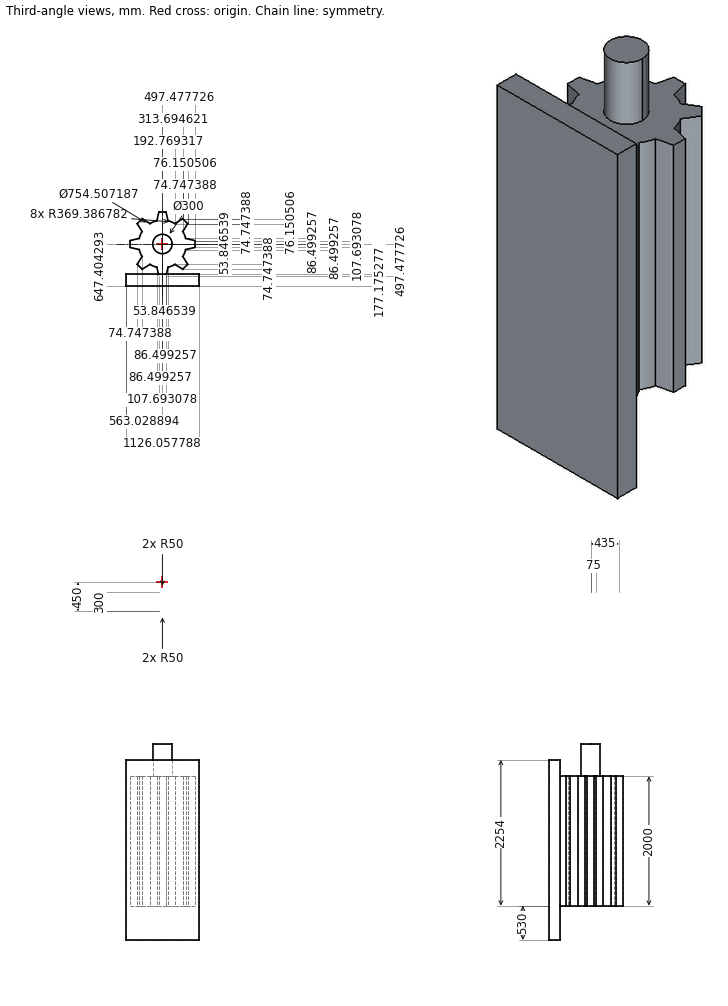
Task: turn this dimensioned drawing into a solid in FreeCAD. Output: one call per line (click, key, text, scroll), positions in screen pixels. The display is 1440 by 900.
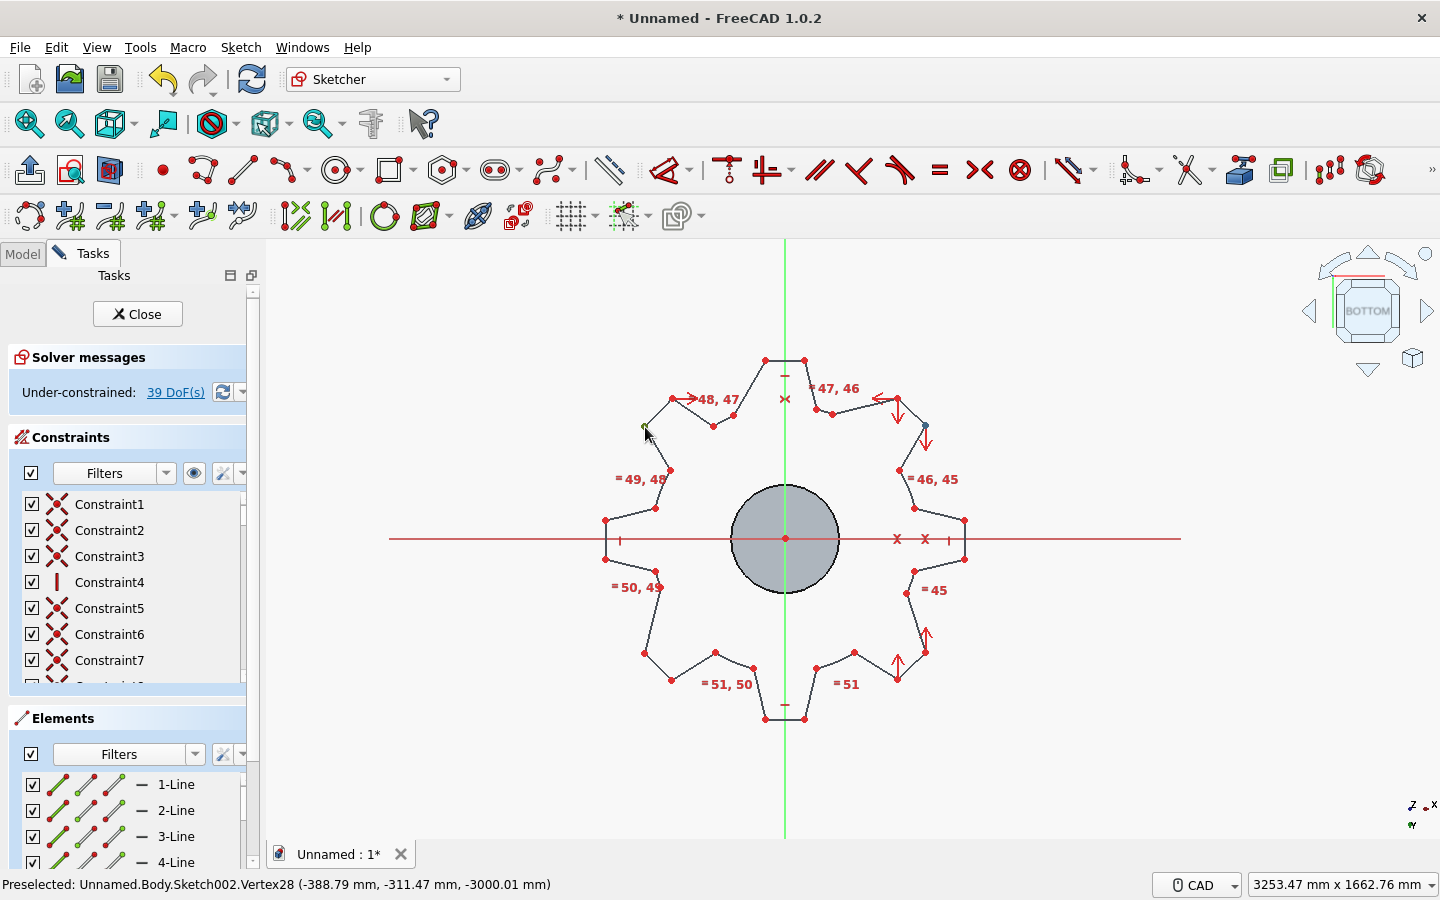
click(785, 772)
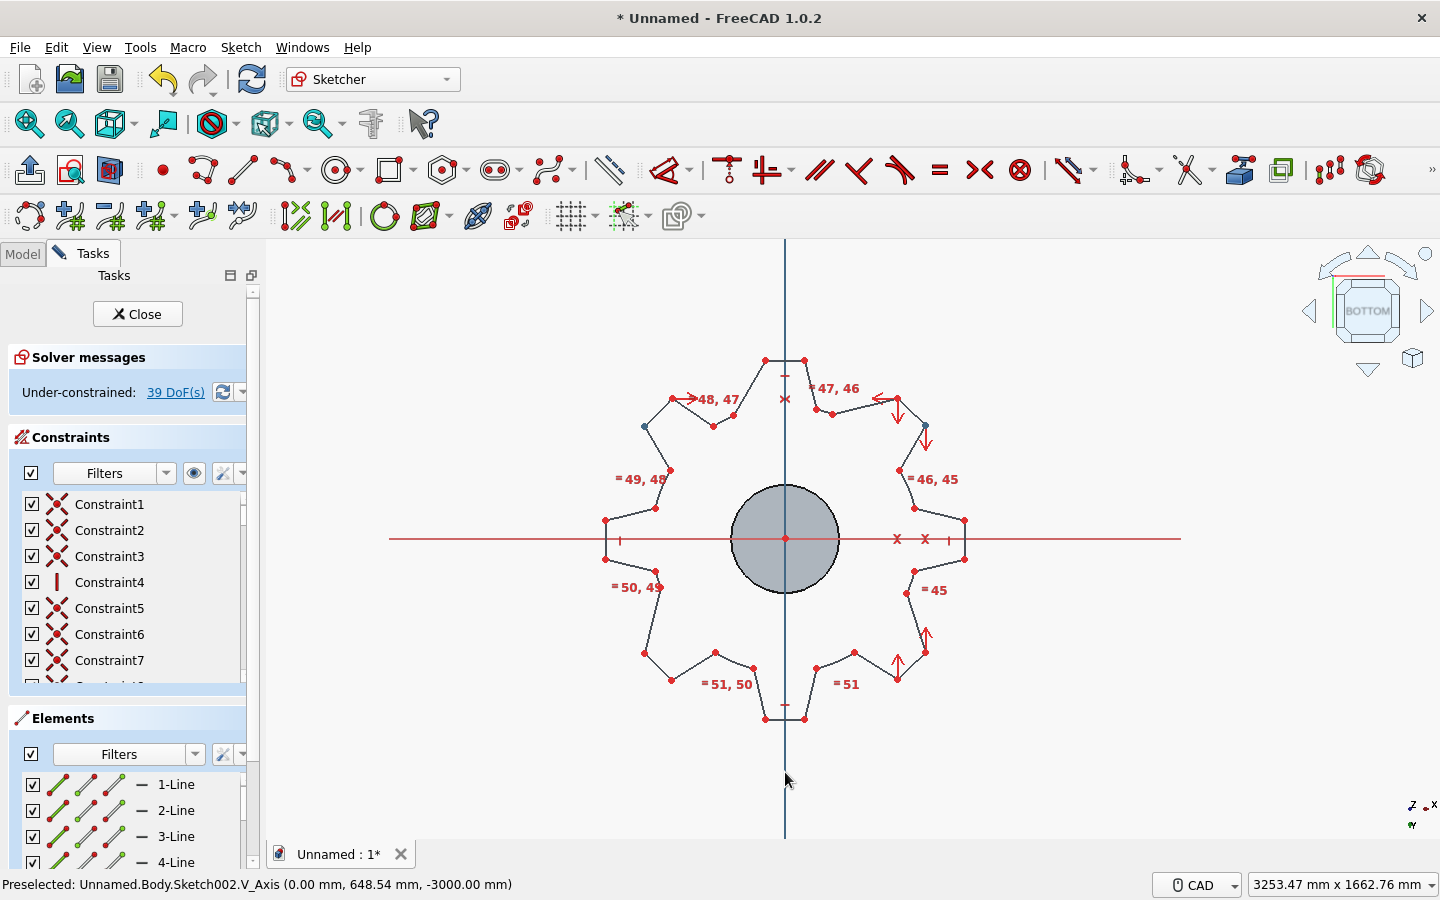
click(980, 170)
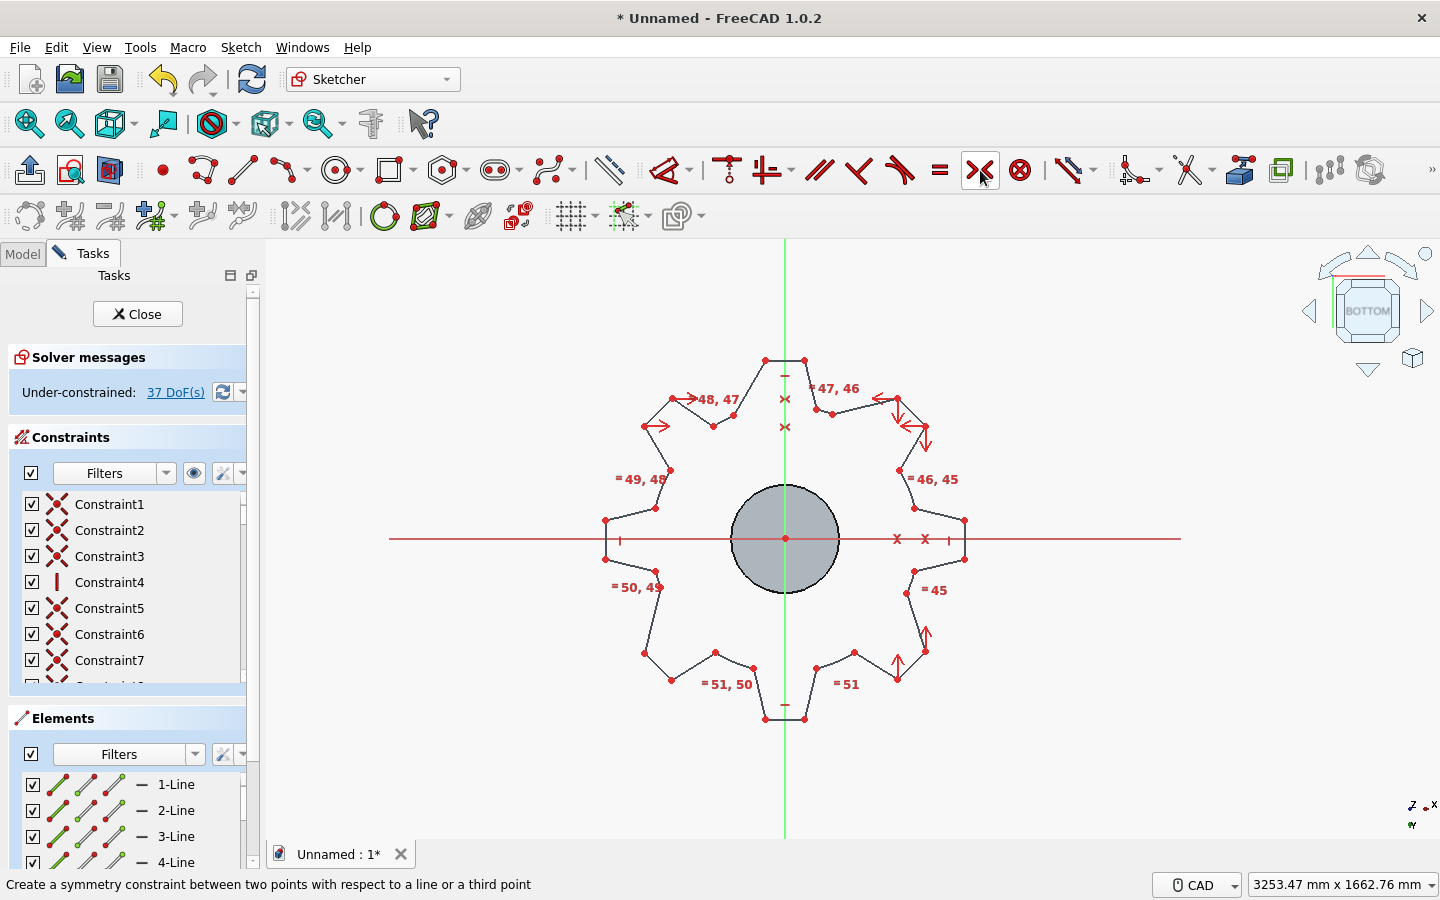
click(965, 521)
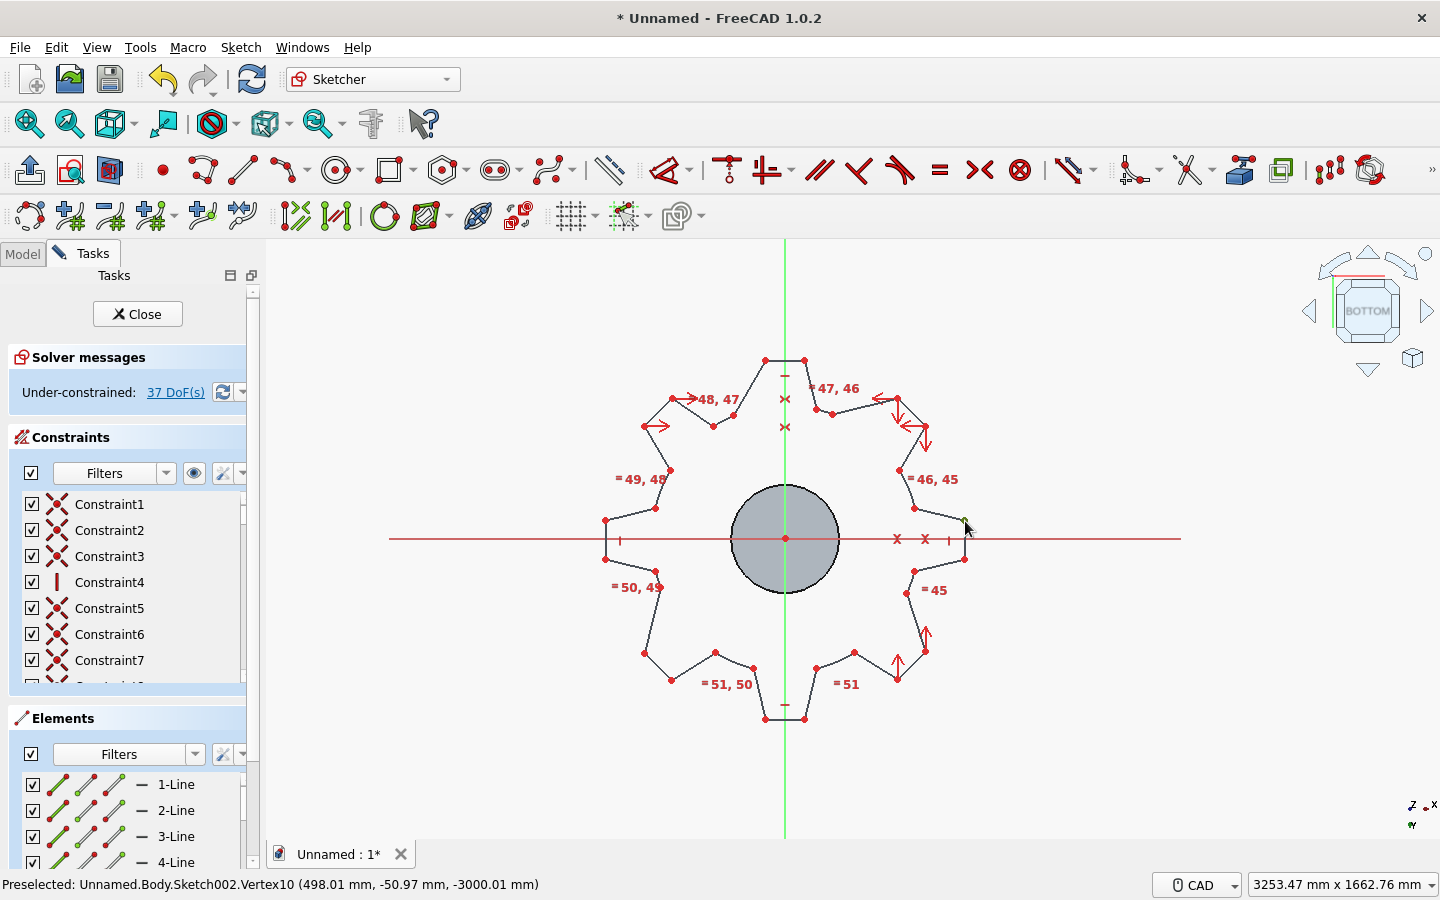
click(606, 521)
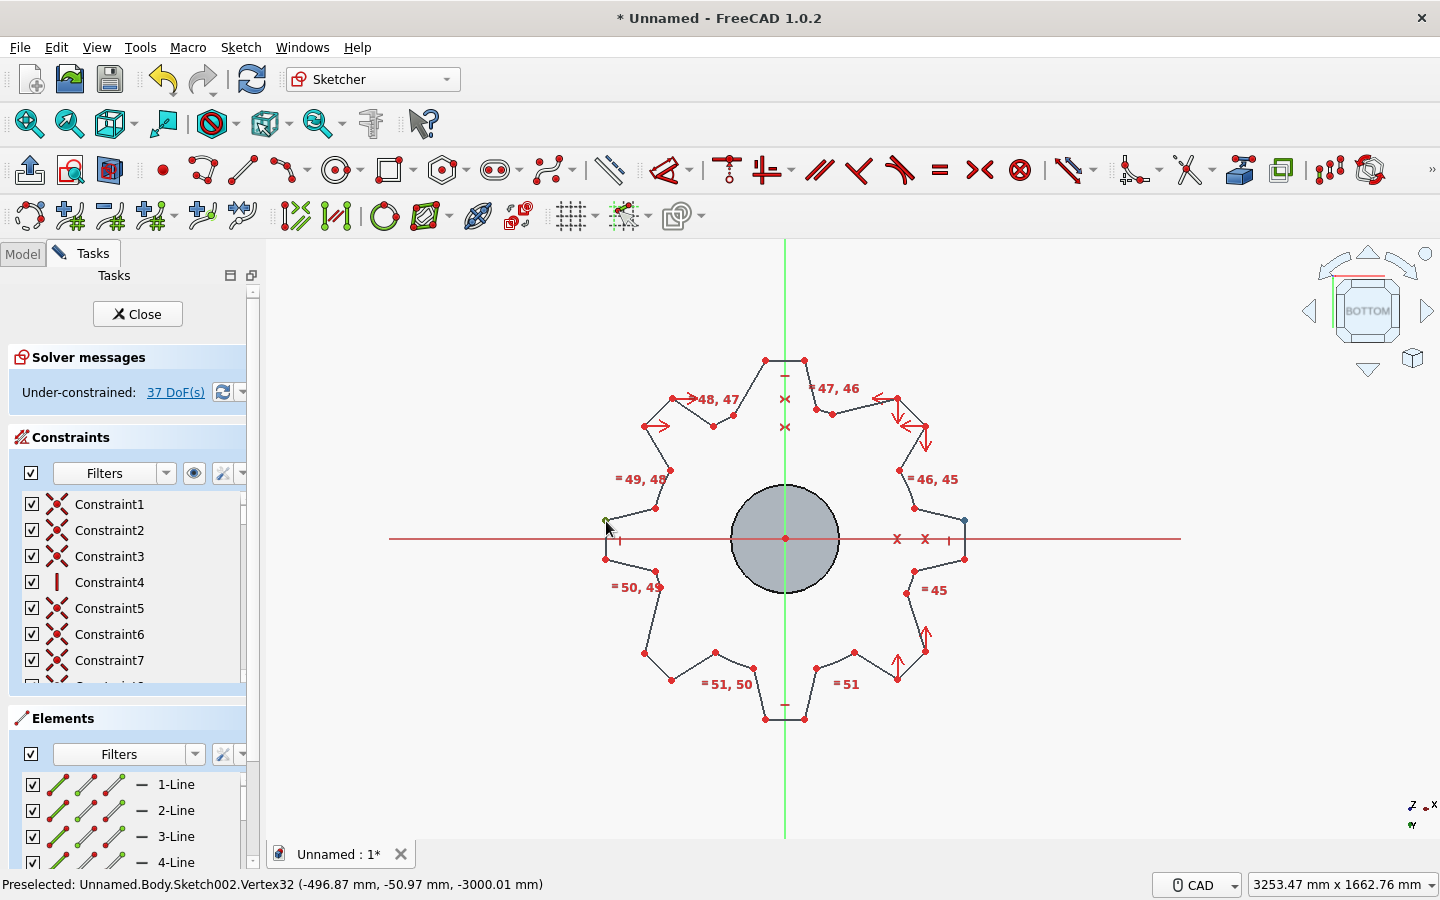
click(785, 772)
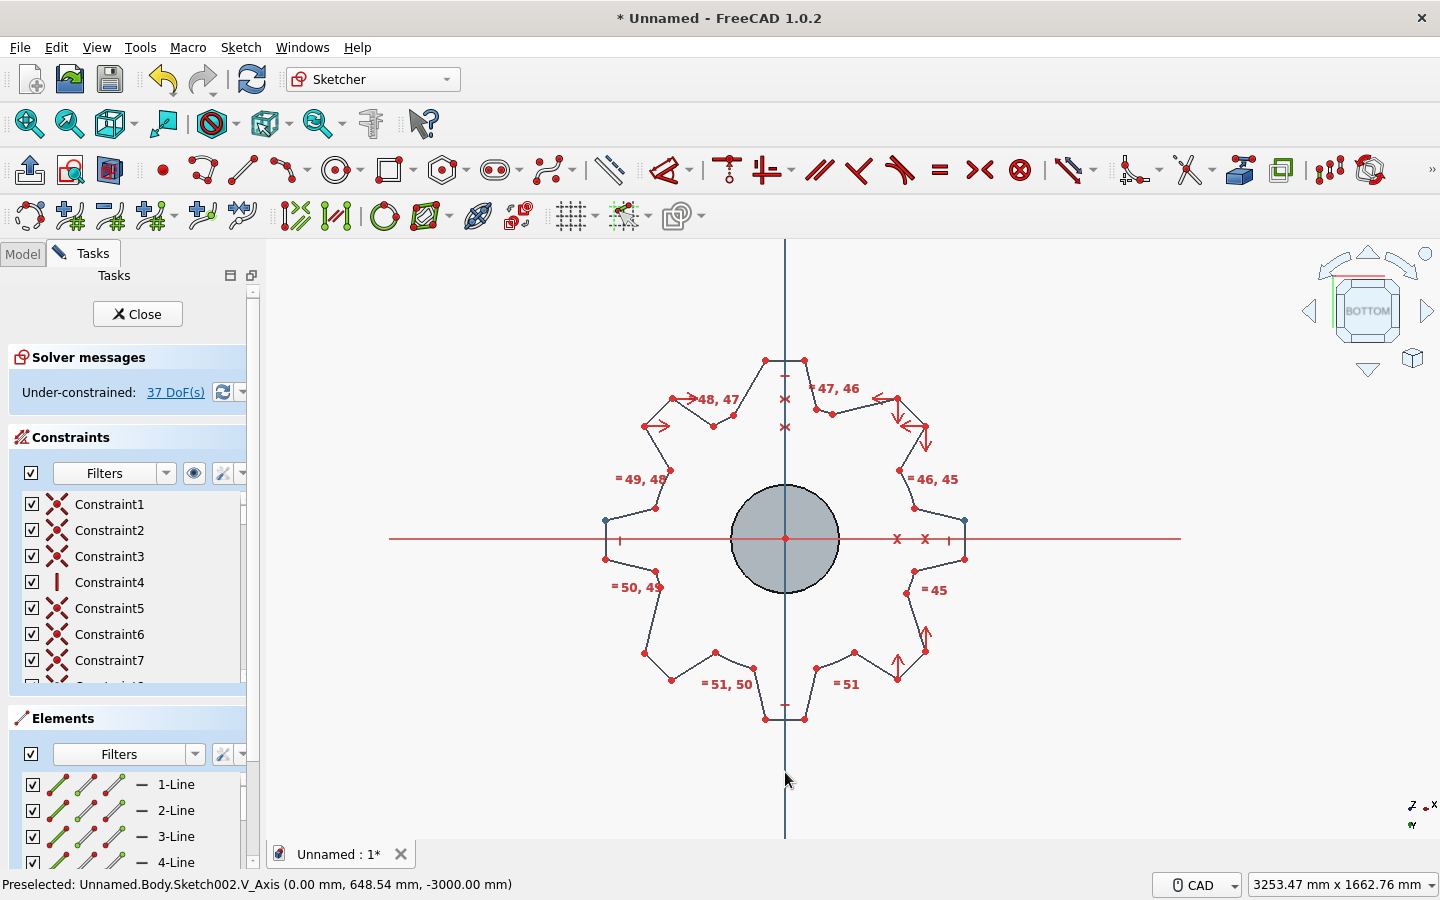
click(980, 170)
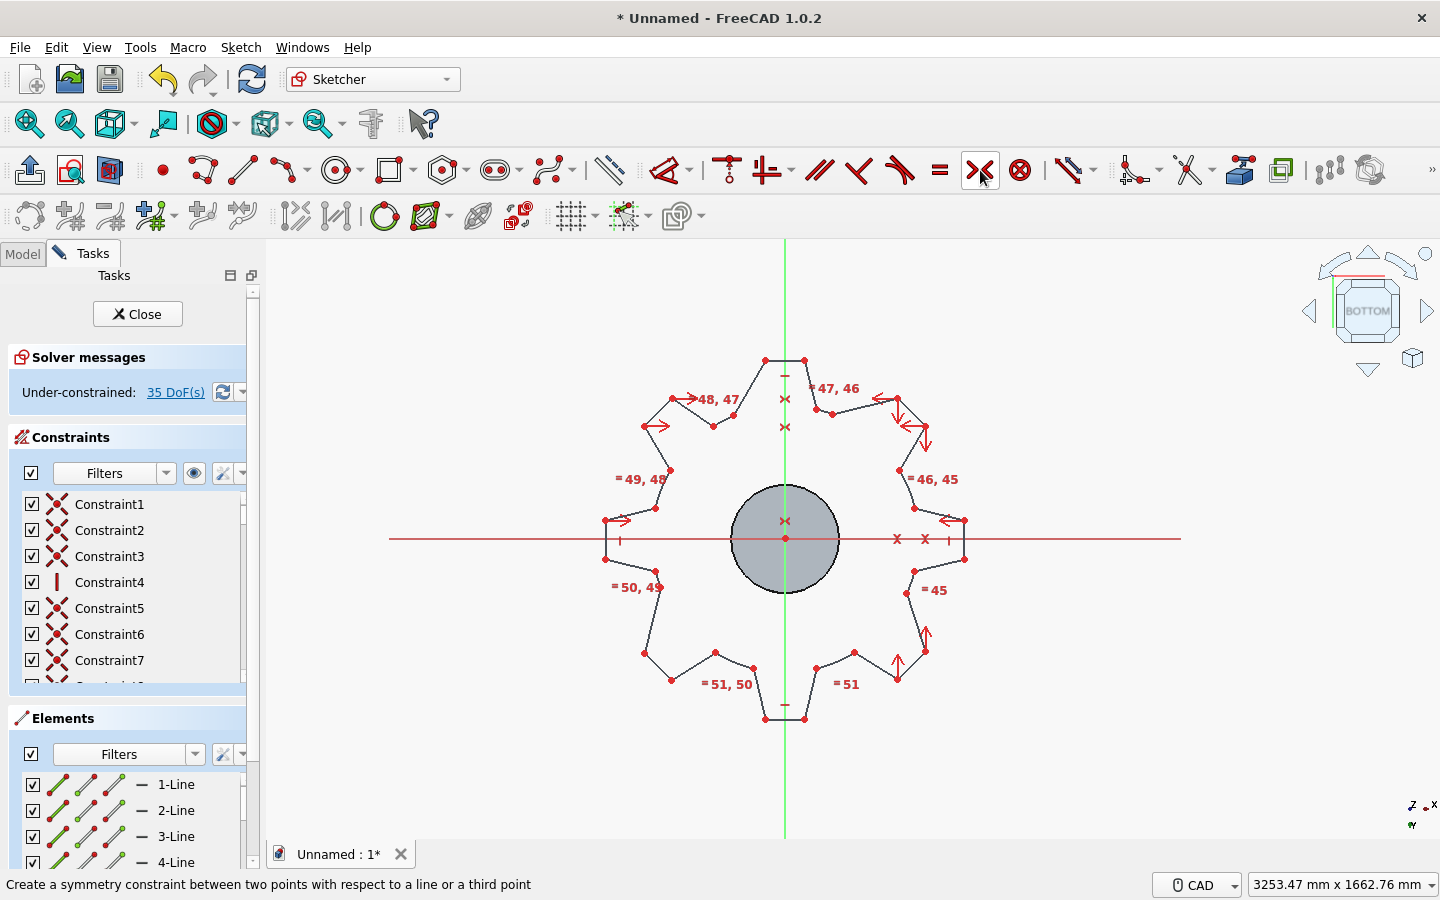
click(926, 652)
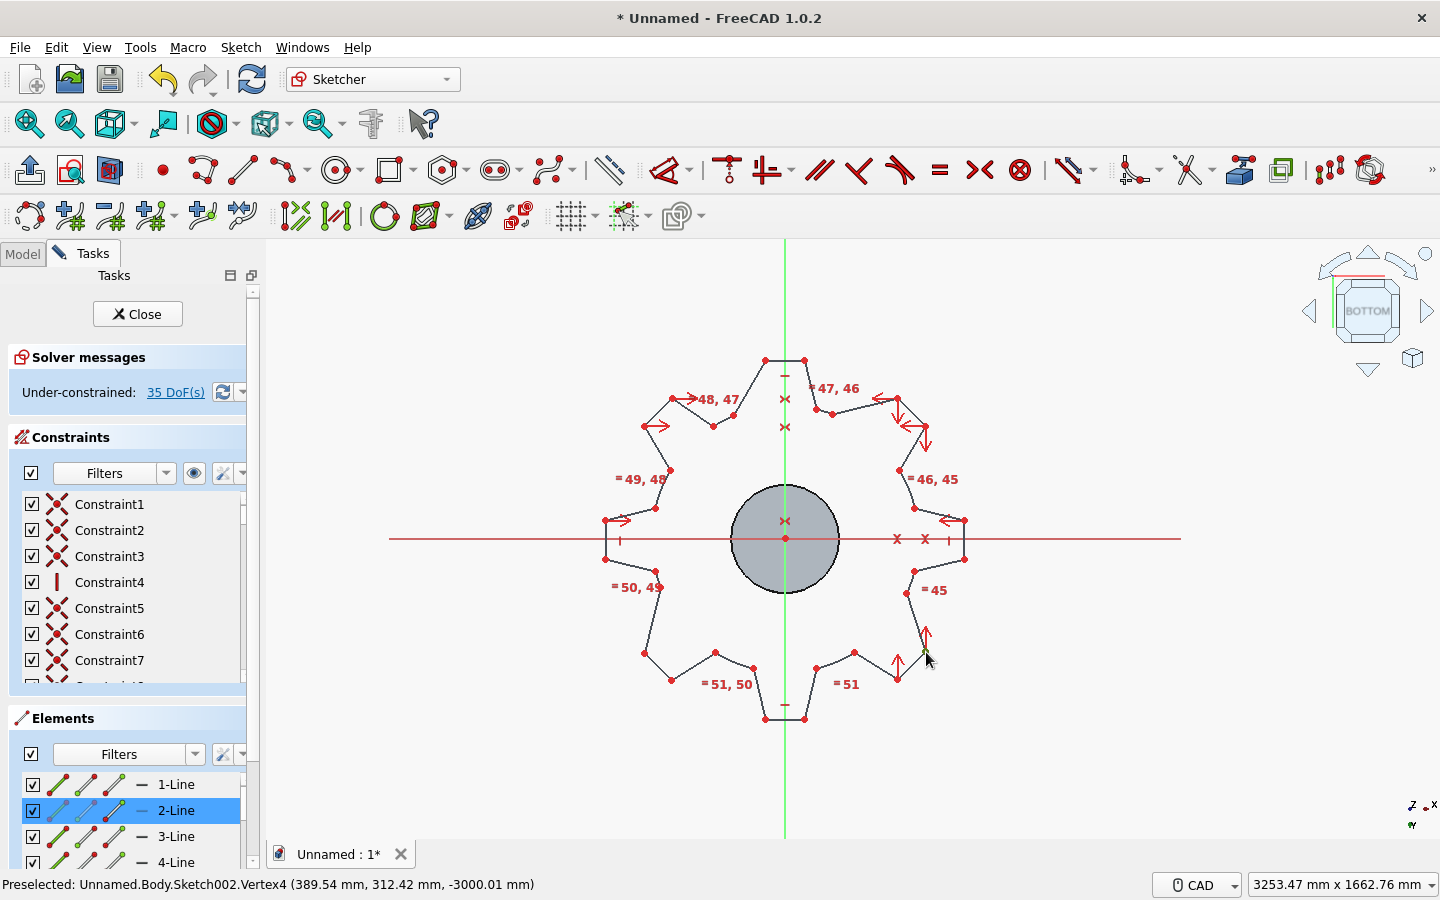
click(645, 654)